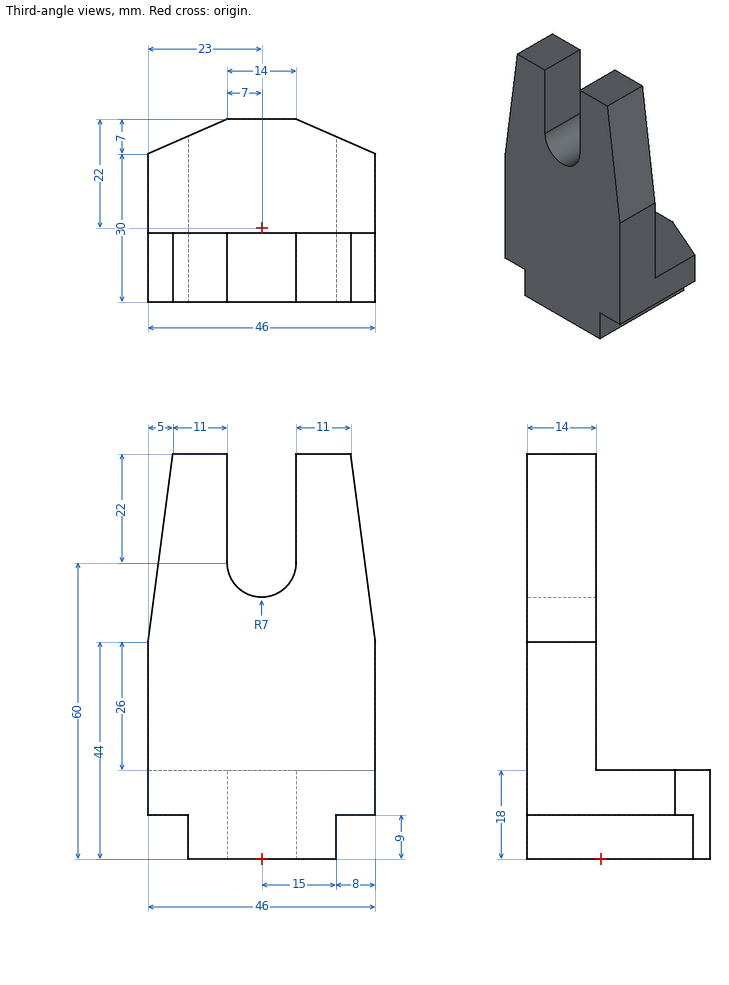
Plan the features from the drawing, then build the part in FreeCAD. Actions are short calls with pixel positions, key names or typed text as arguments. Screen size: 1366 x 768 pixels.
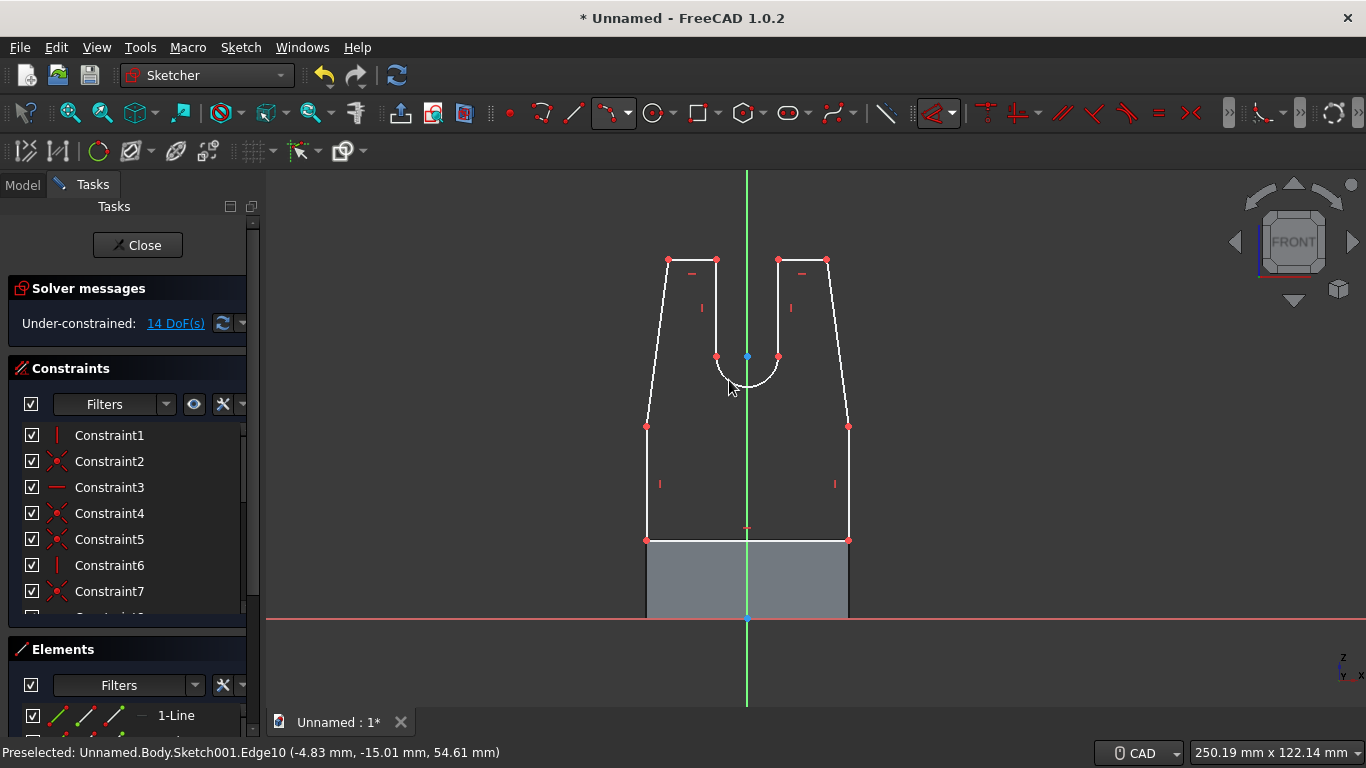
click(716, 327)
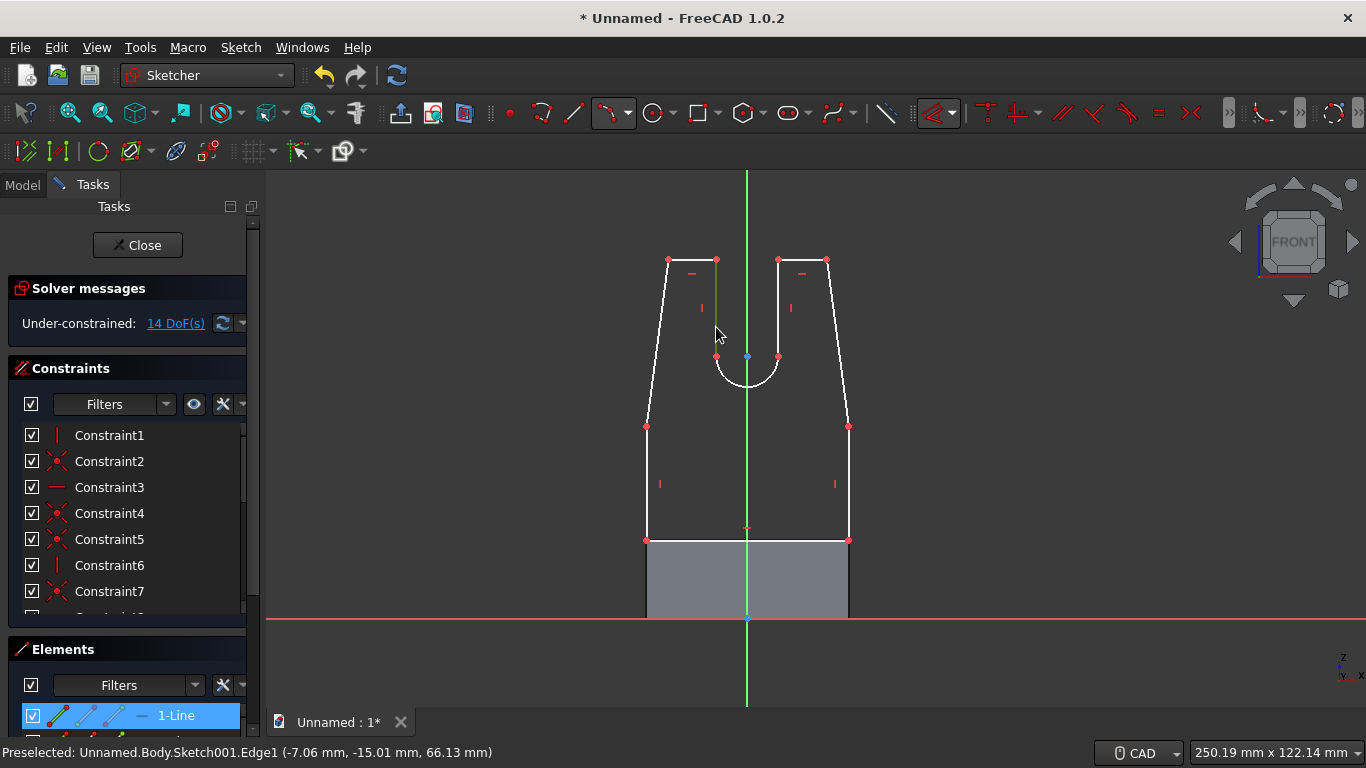
click(729, 381)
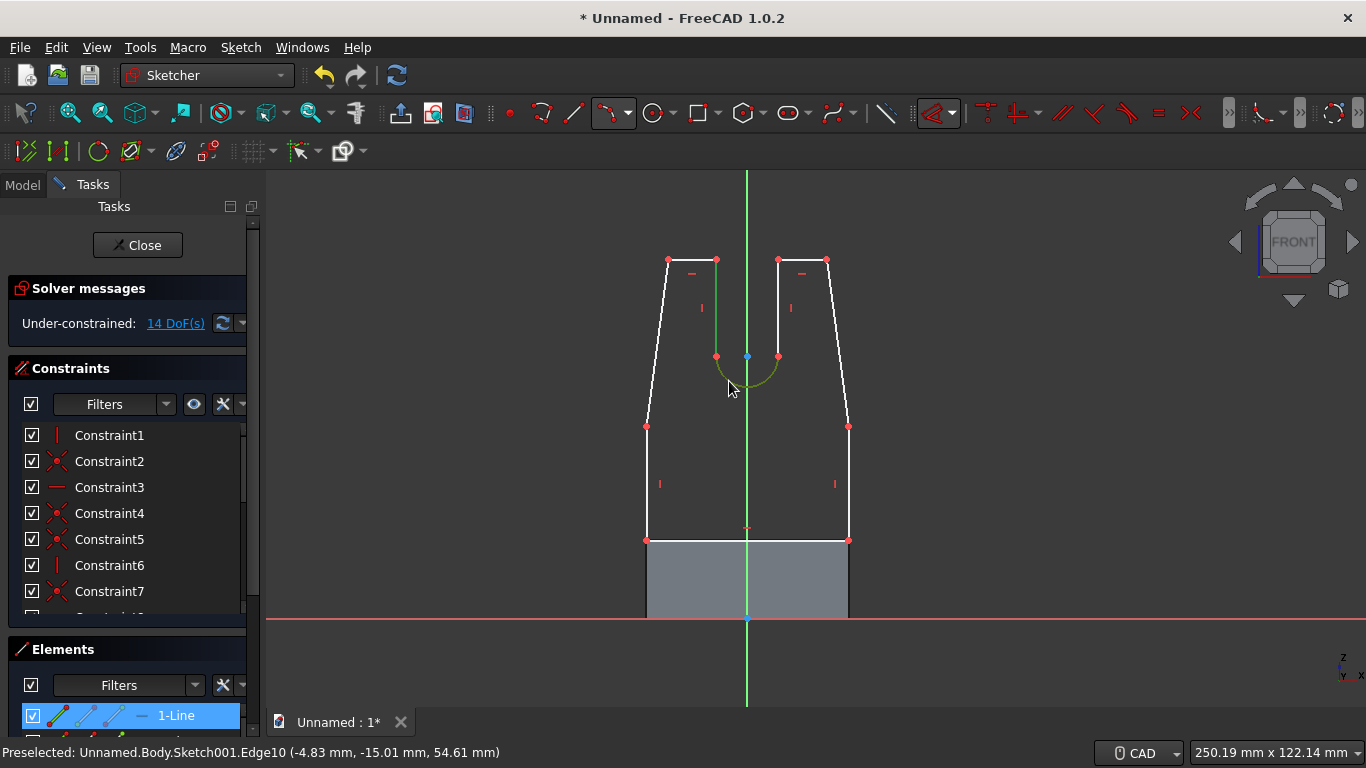
click(1128, 114)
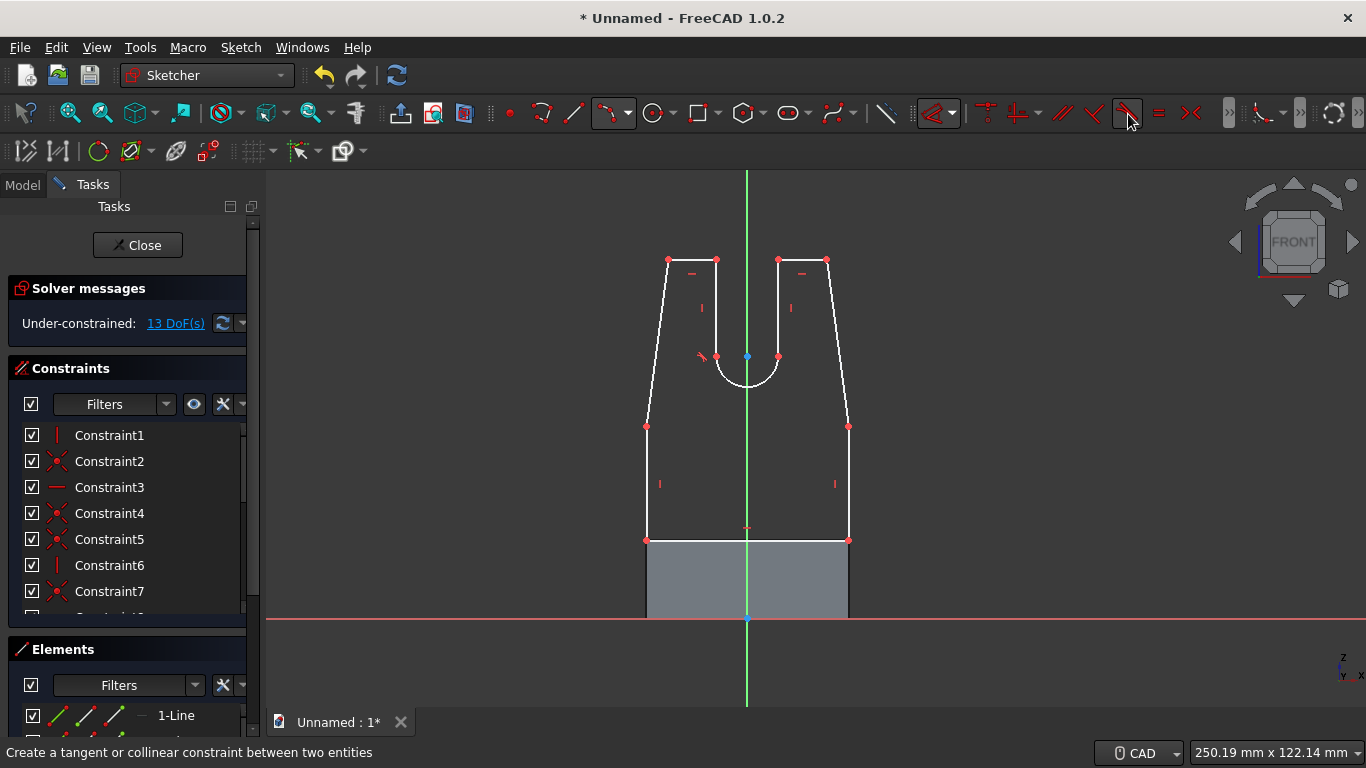
click(778, 289)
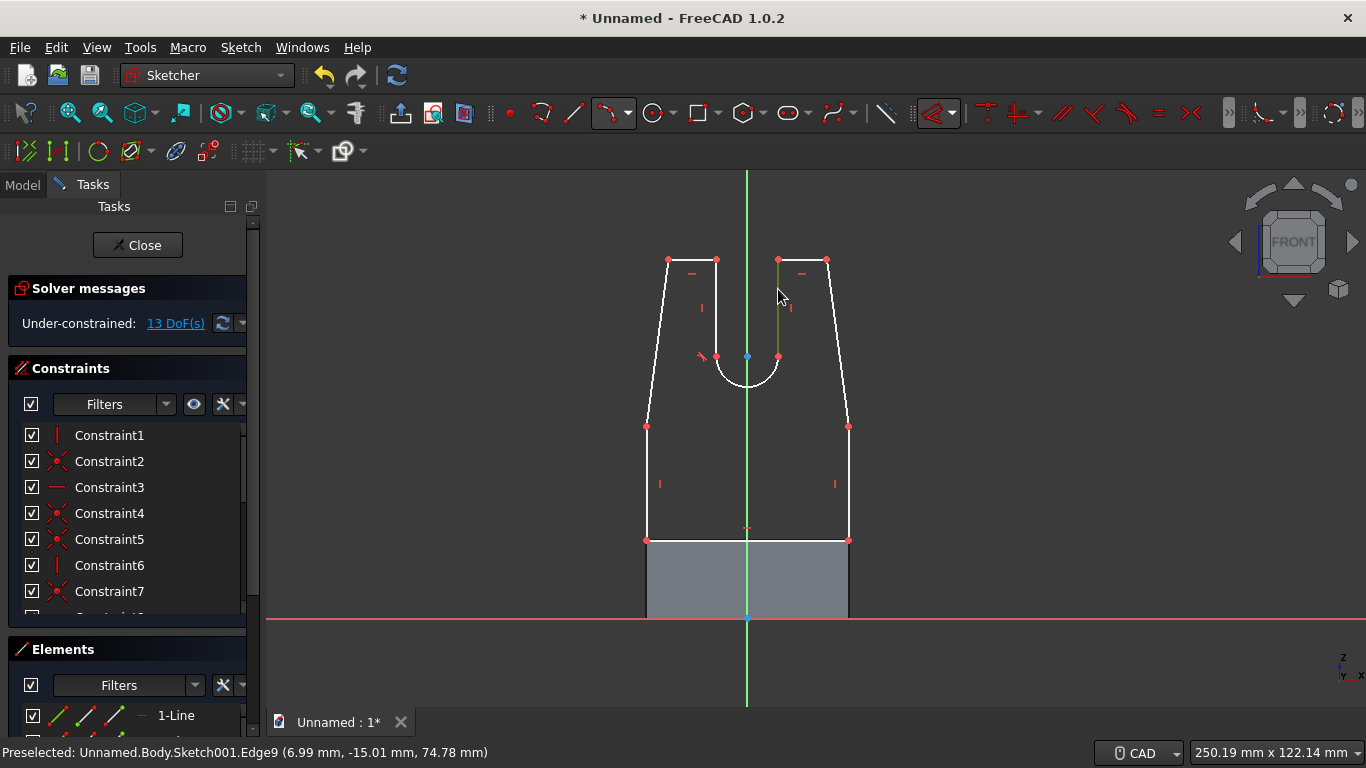
click(729, 381)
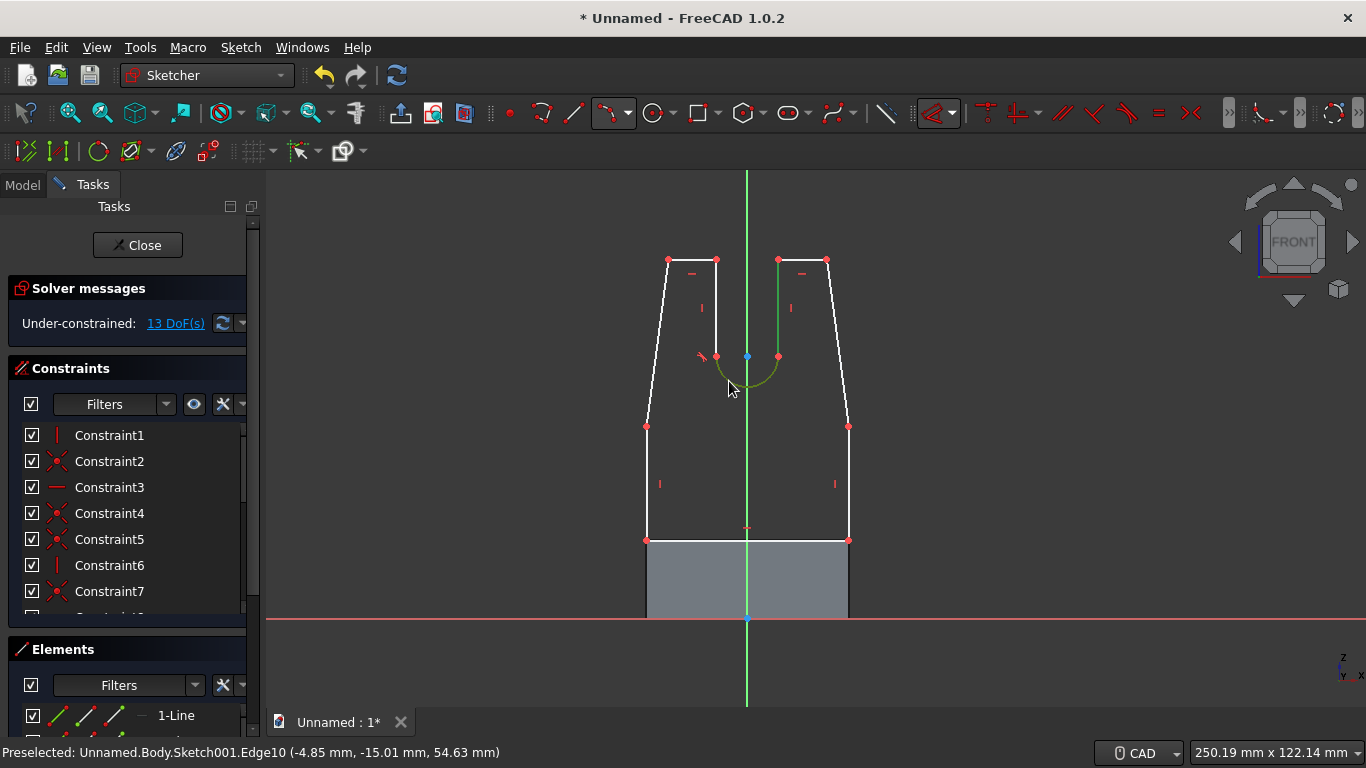
click(1128, 114)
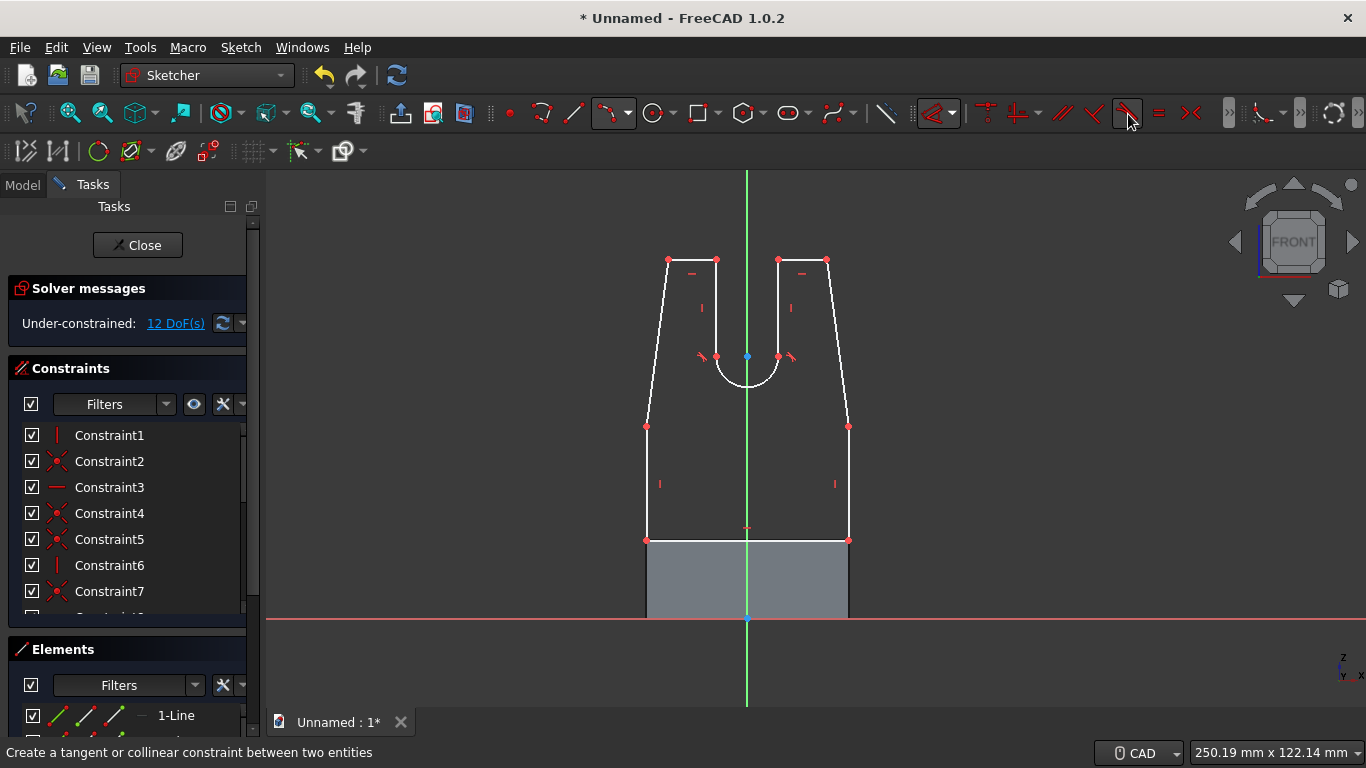
click(747, 356)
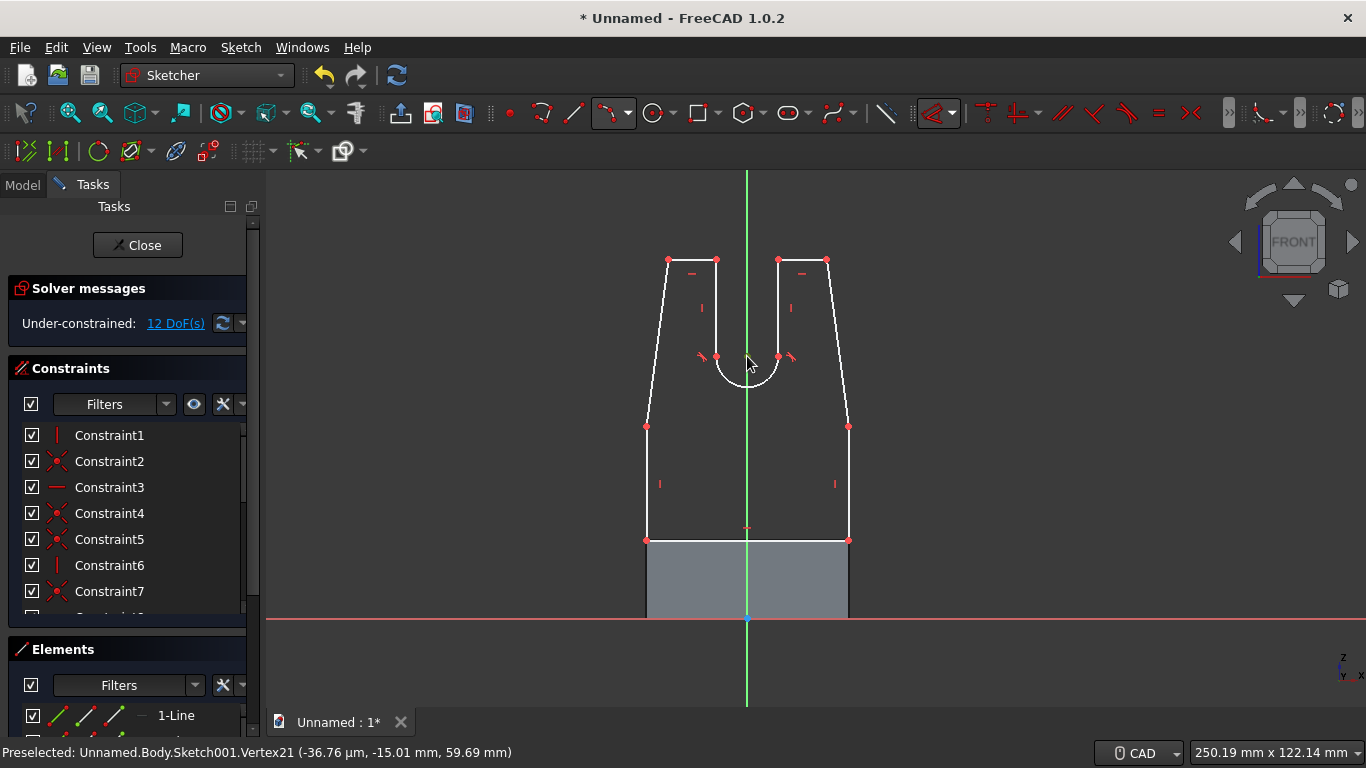
click(747, 576)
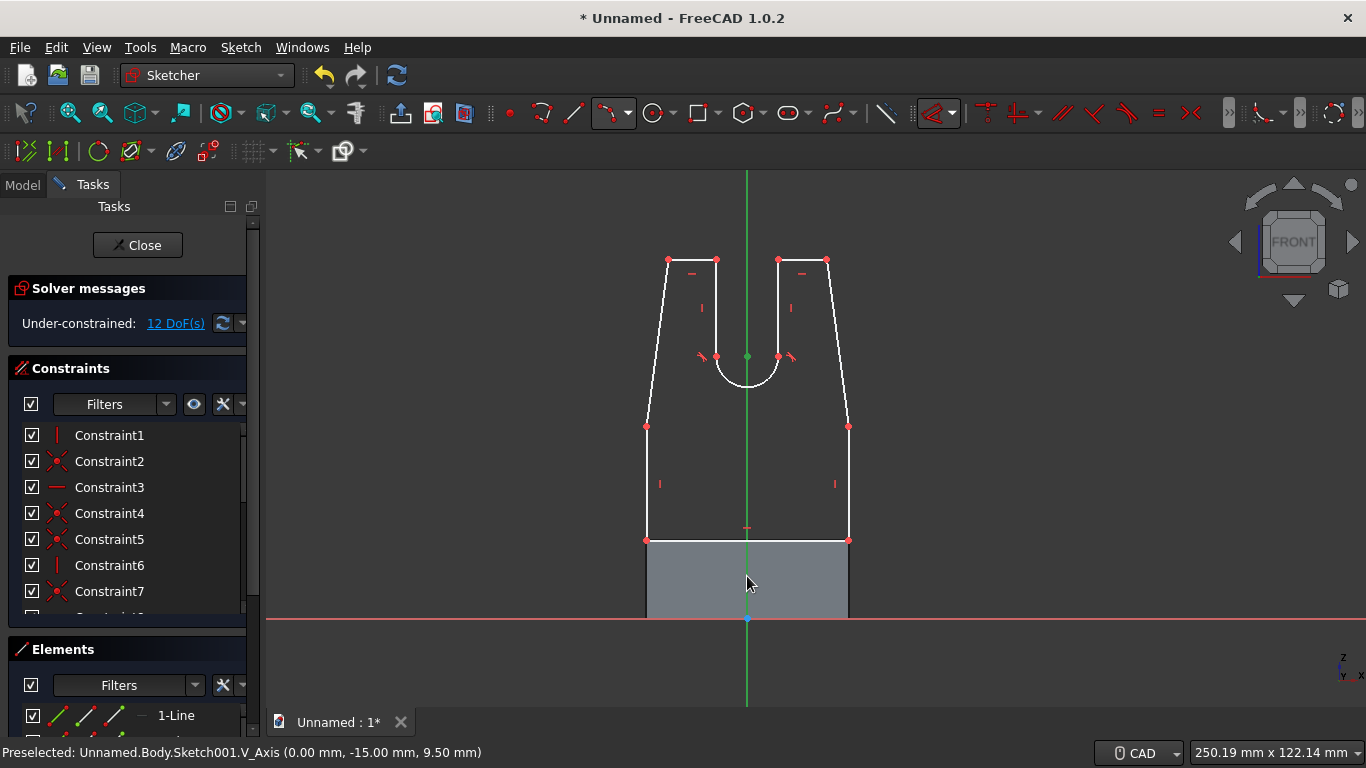
click(986, 114)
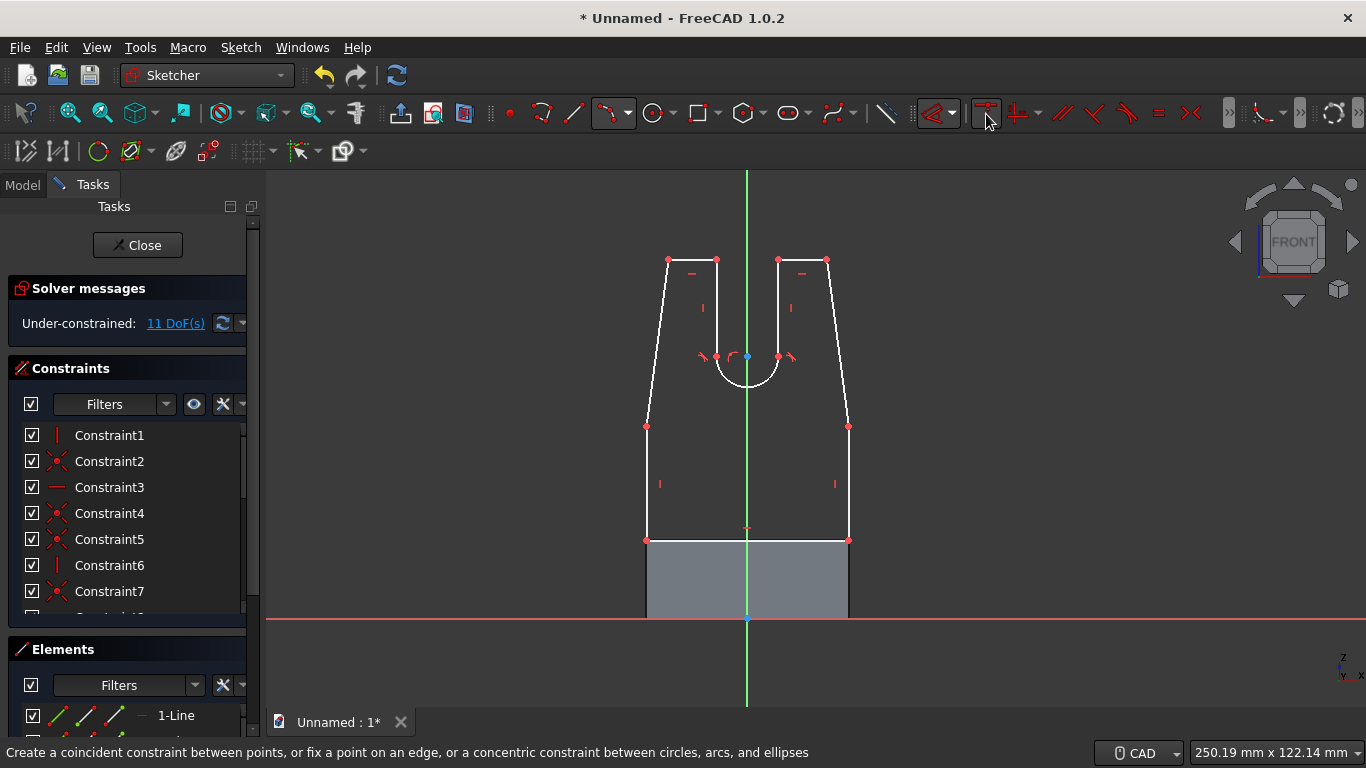
scroll(729, 381, up, 2)